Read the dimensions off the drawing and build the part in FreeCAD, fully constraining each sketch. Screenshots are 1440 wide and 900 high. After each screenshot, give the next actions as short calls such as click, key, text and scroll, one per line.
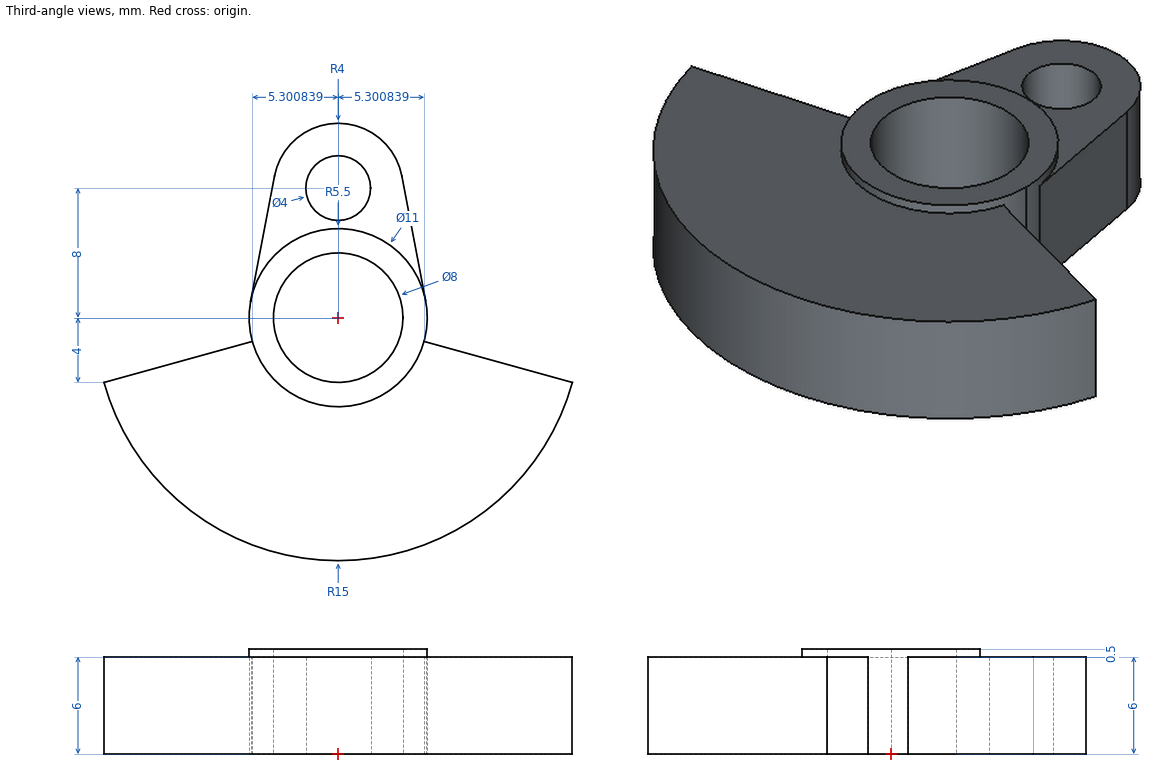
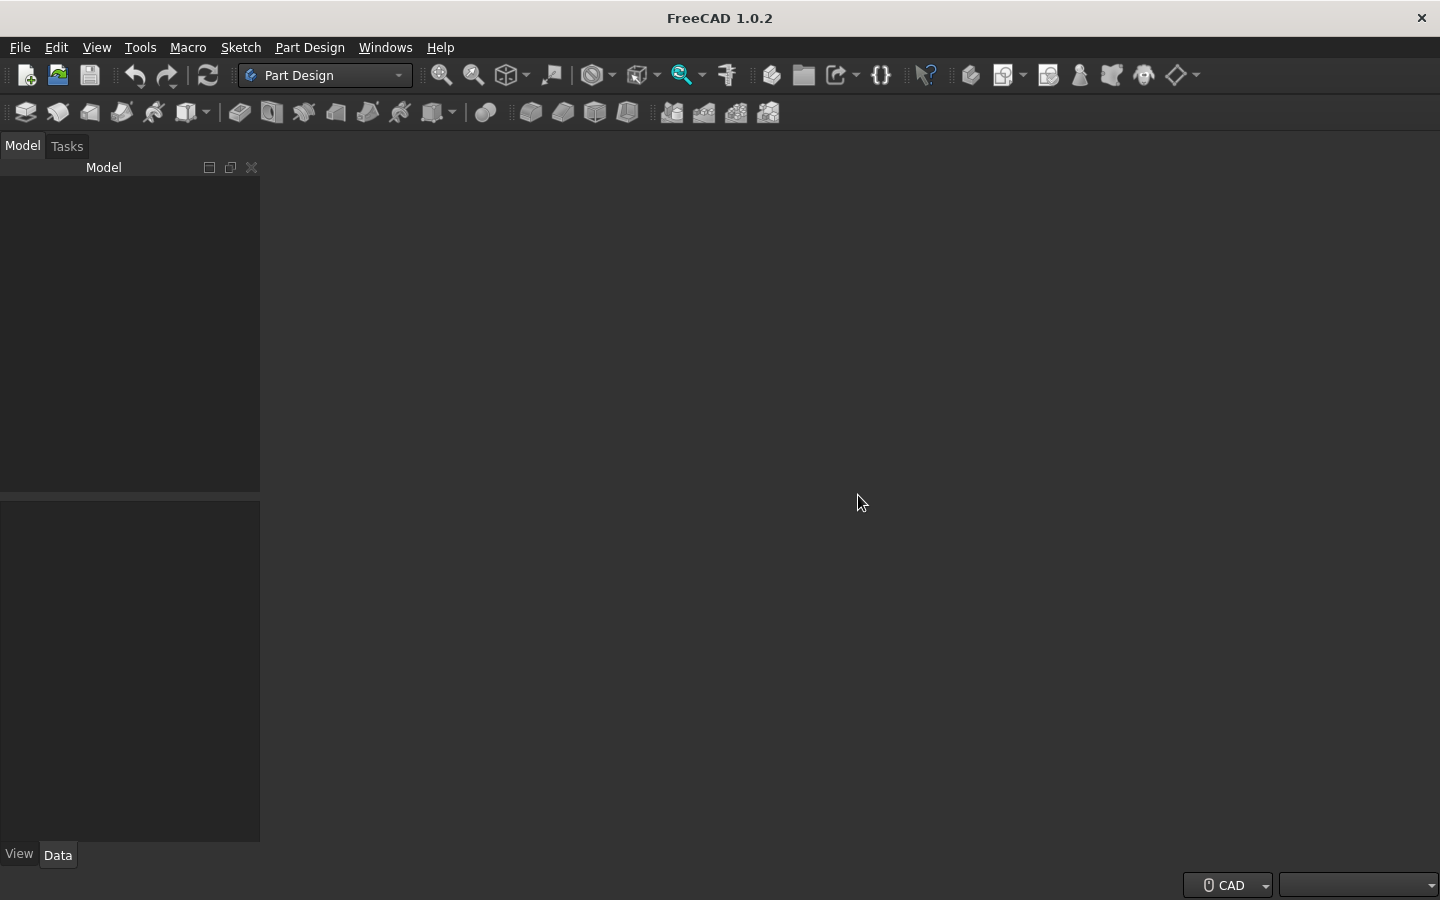
click(26, 76)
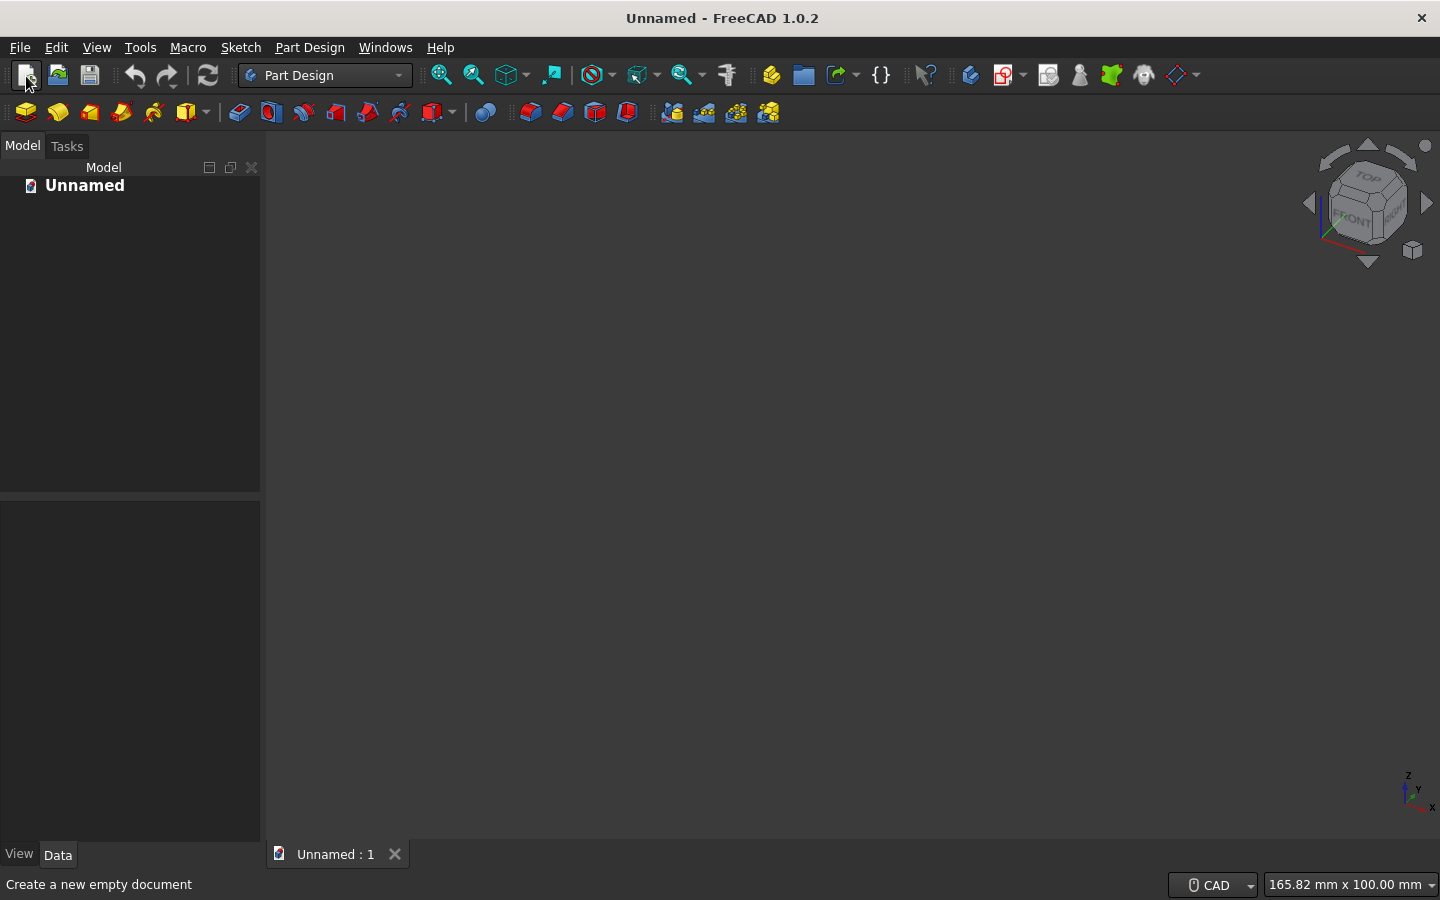
click(1004, 76)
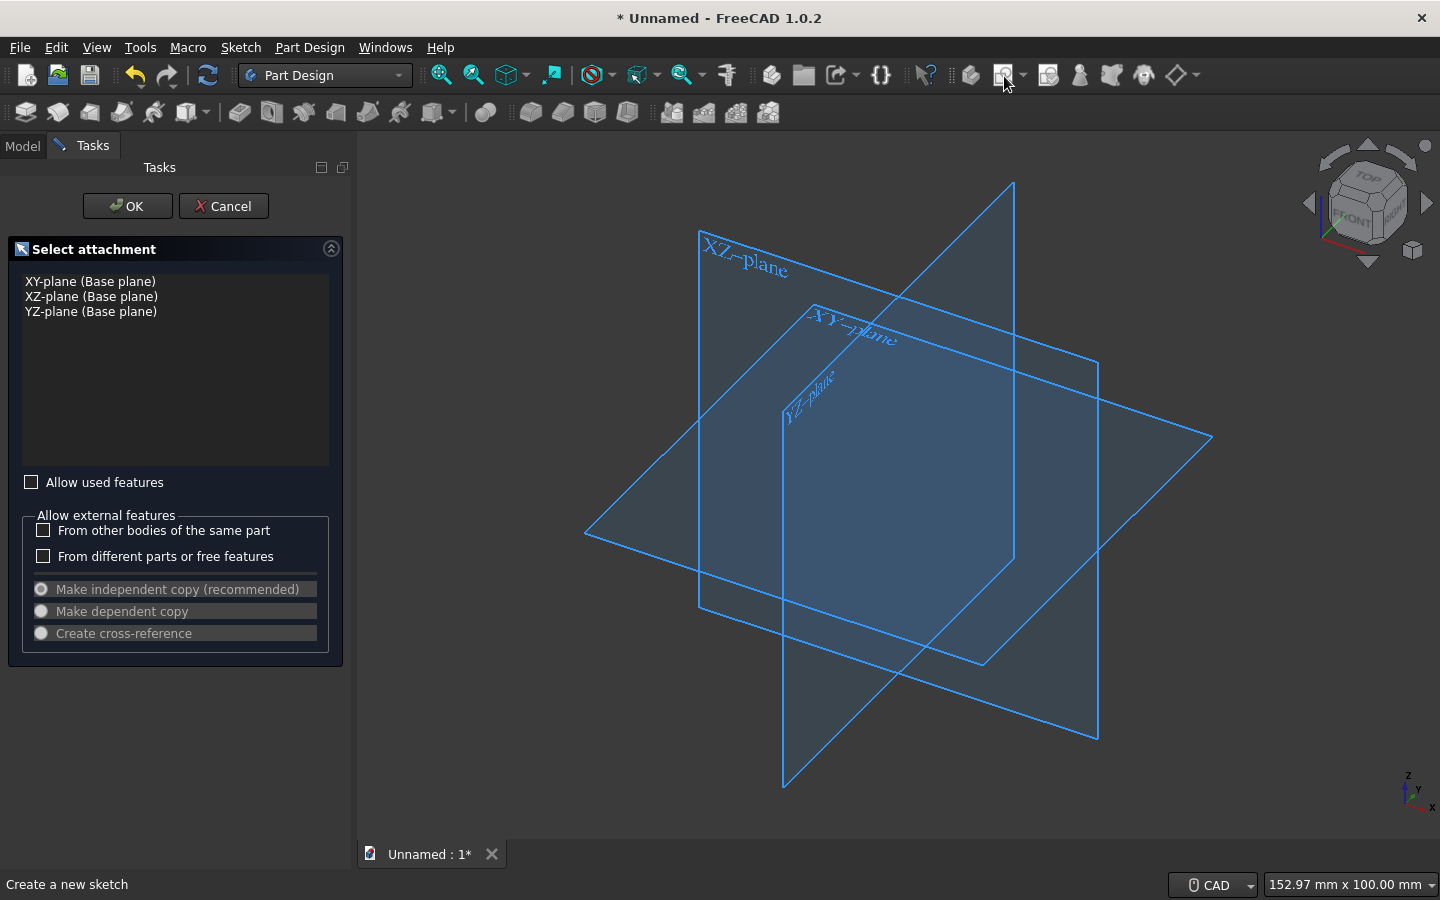
click(82, 282)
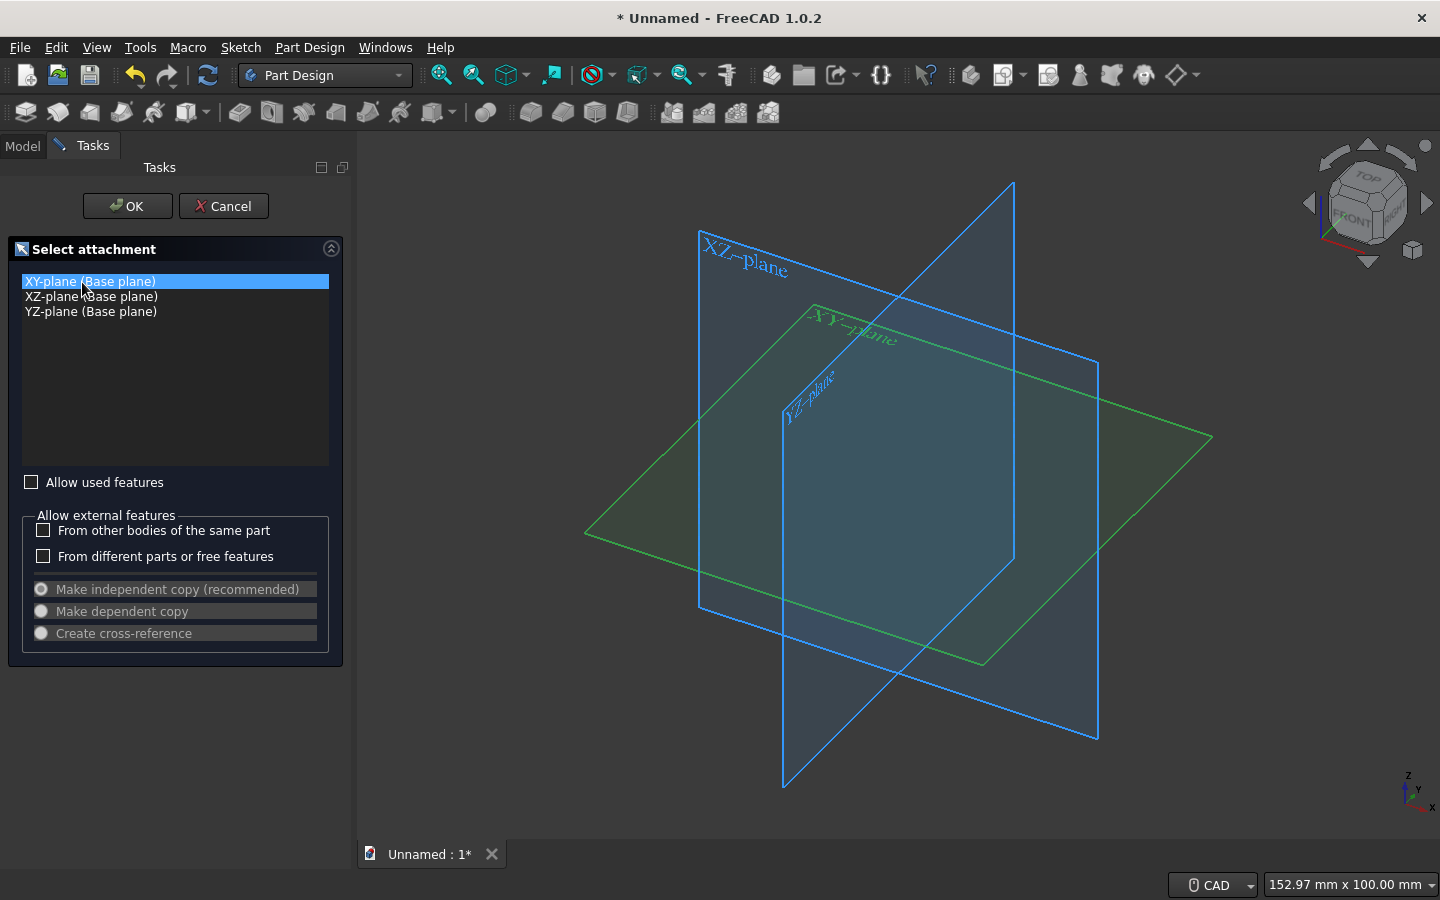
click(128, 206)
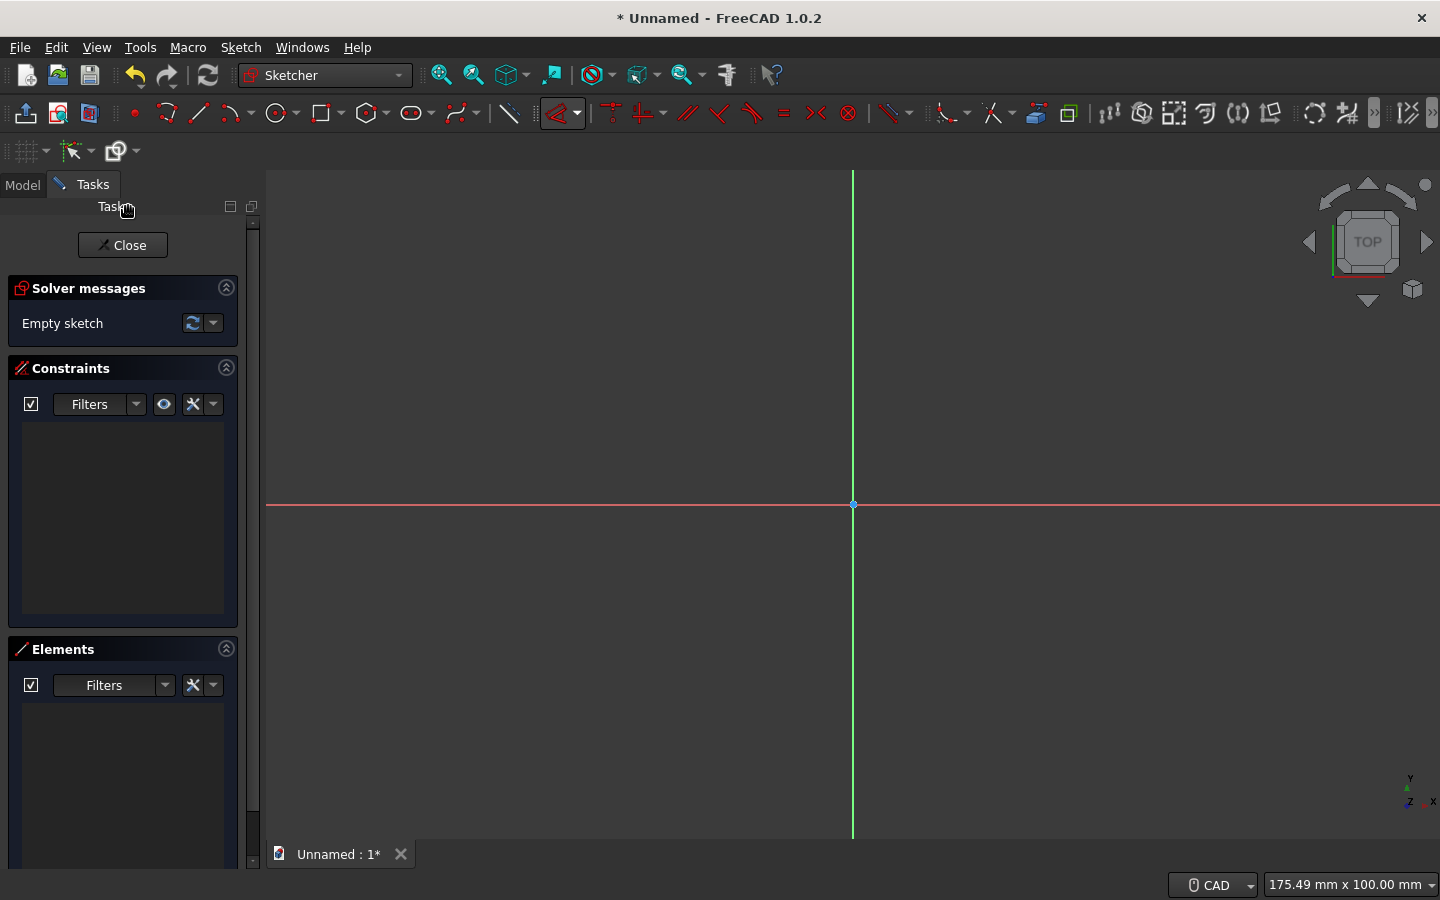
scroll(883, 550, up, 6)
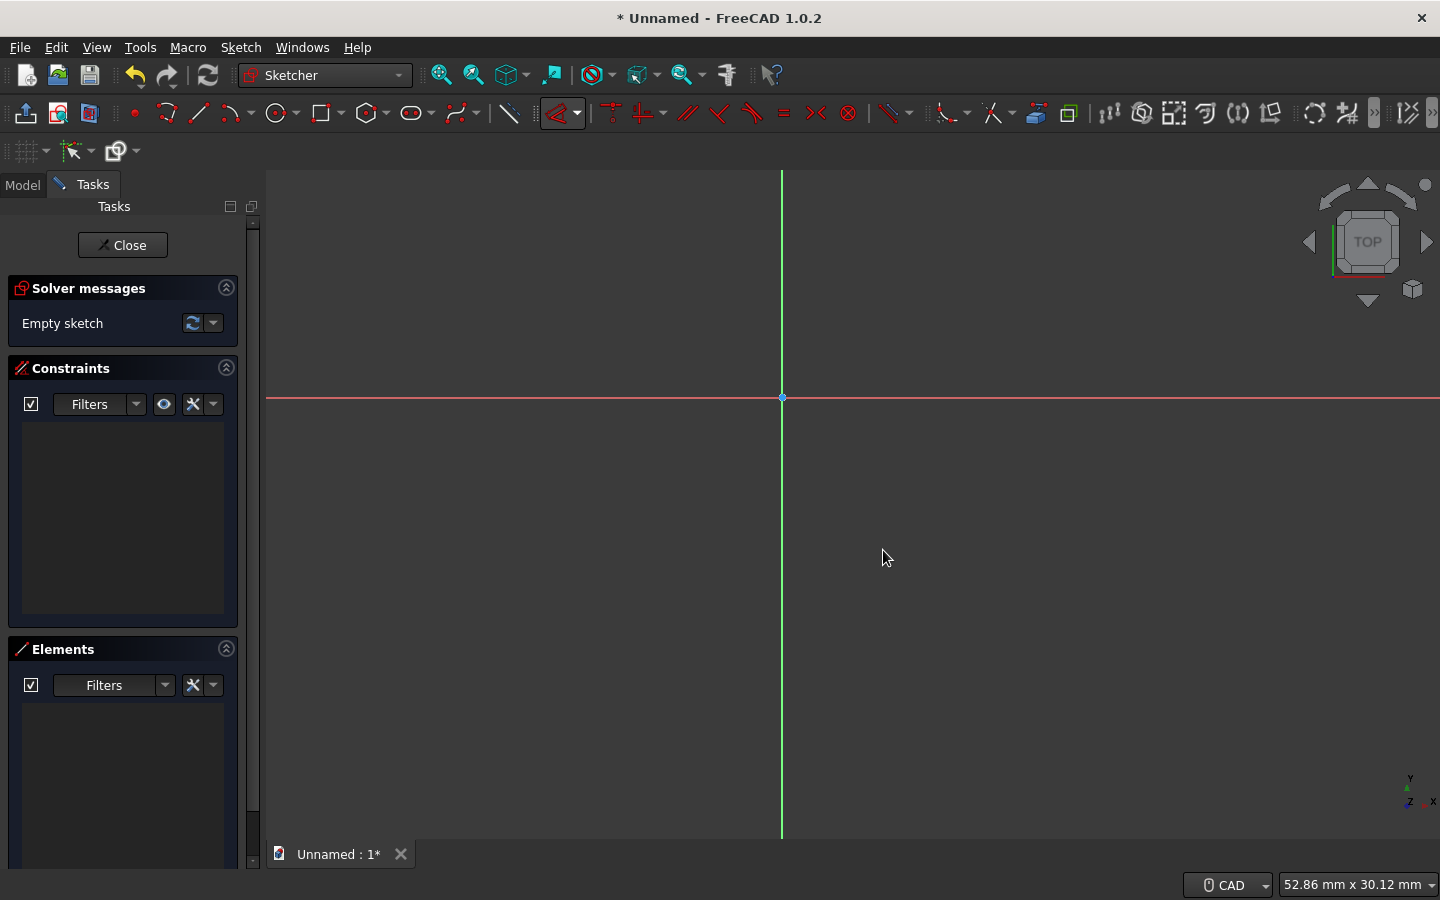
click(200, 114)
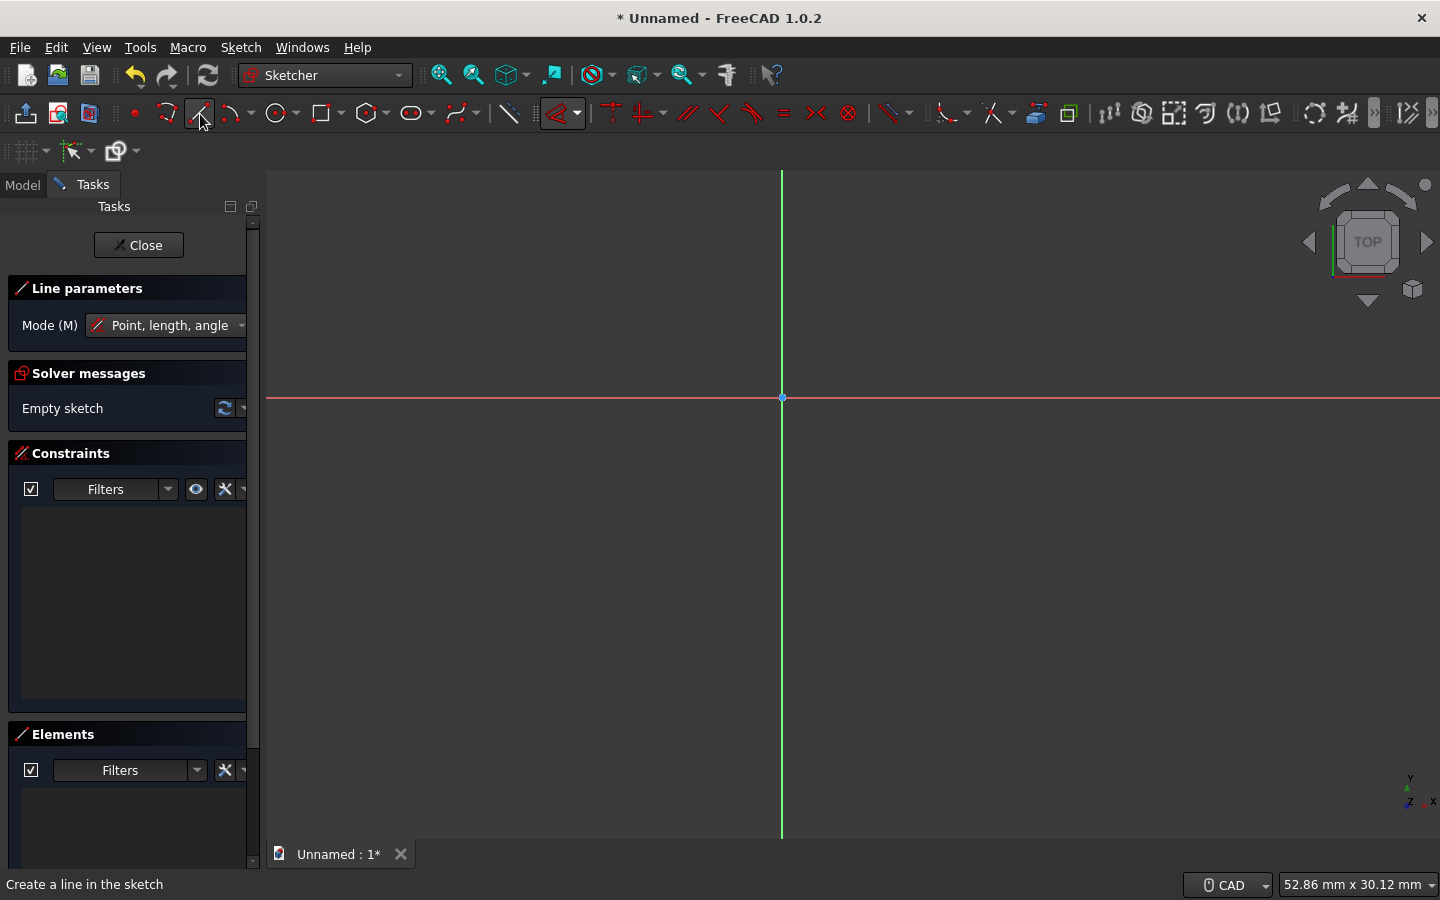
click(664, 430)
click(461, 486)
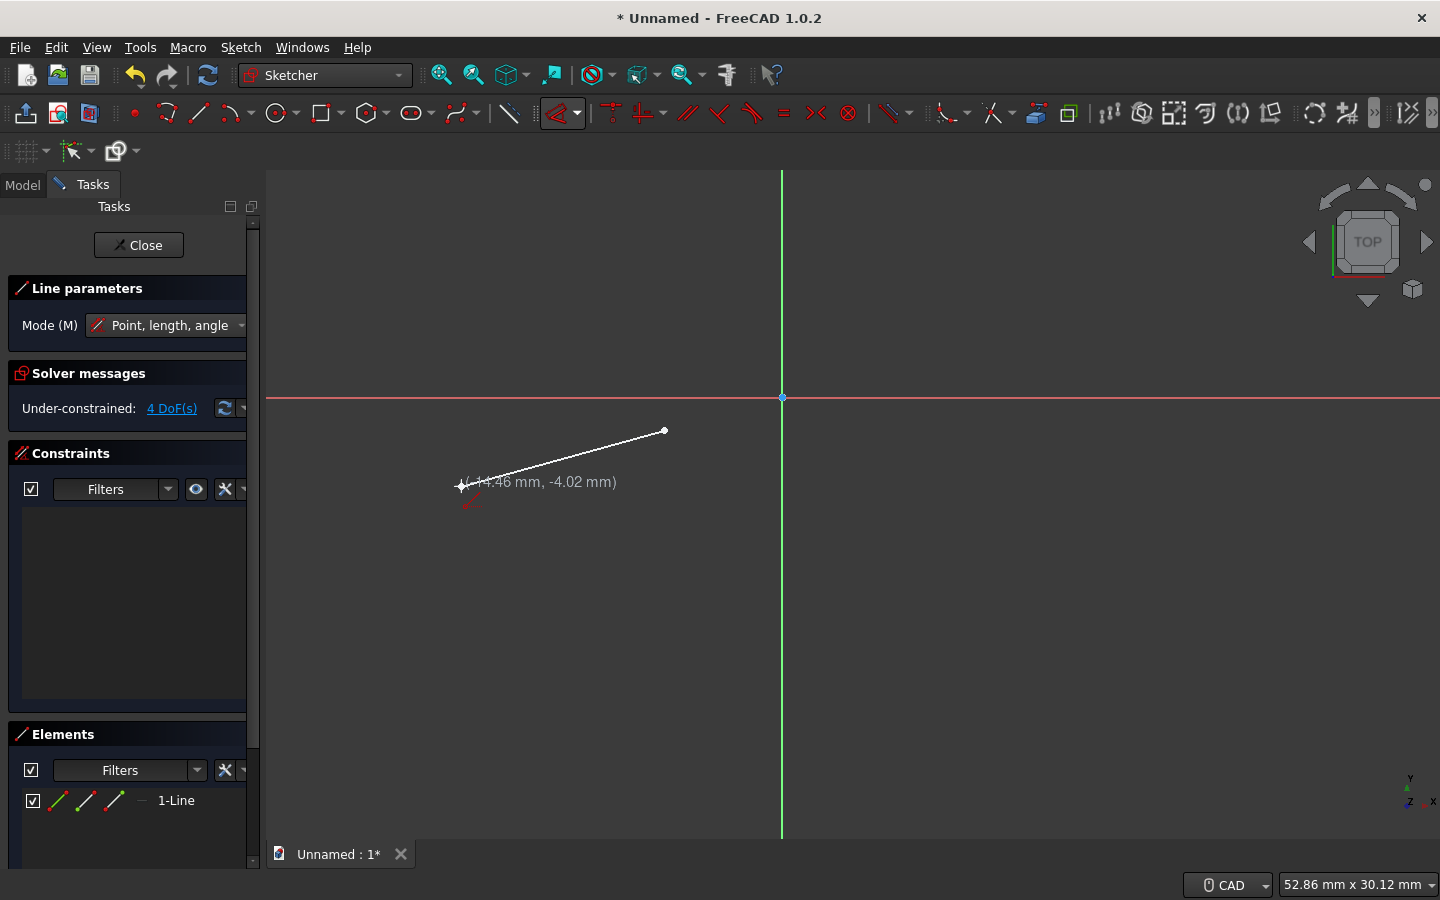
click(1103, 486)
click(900, 430)